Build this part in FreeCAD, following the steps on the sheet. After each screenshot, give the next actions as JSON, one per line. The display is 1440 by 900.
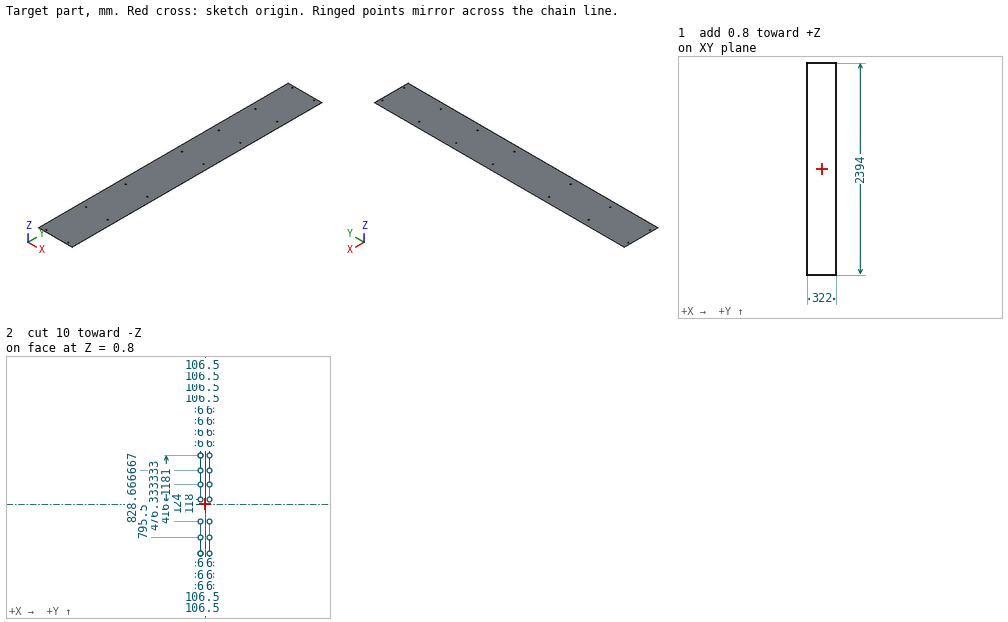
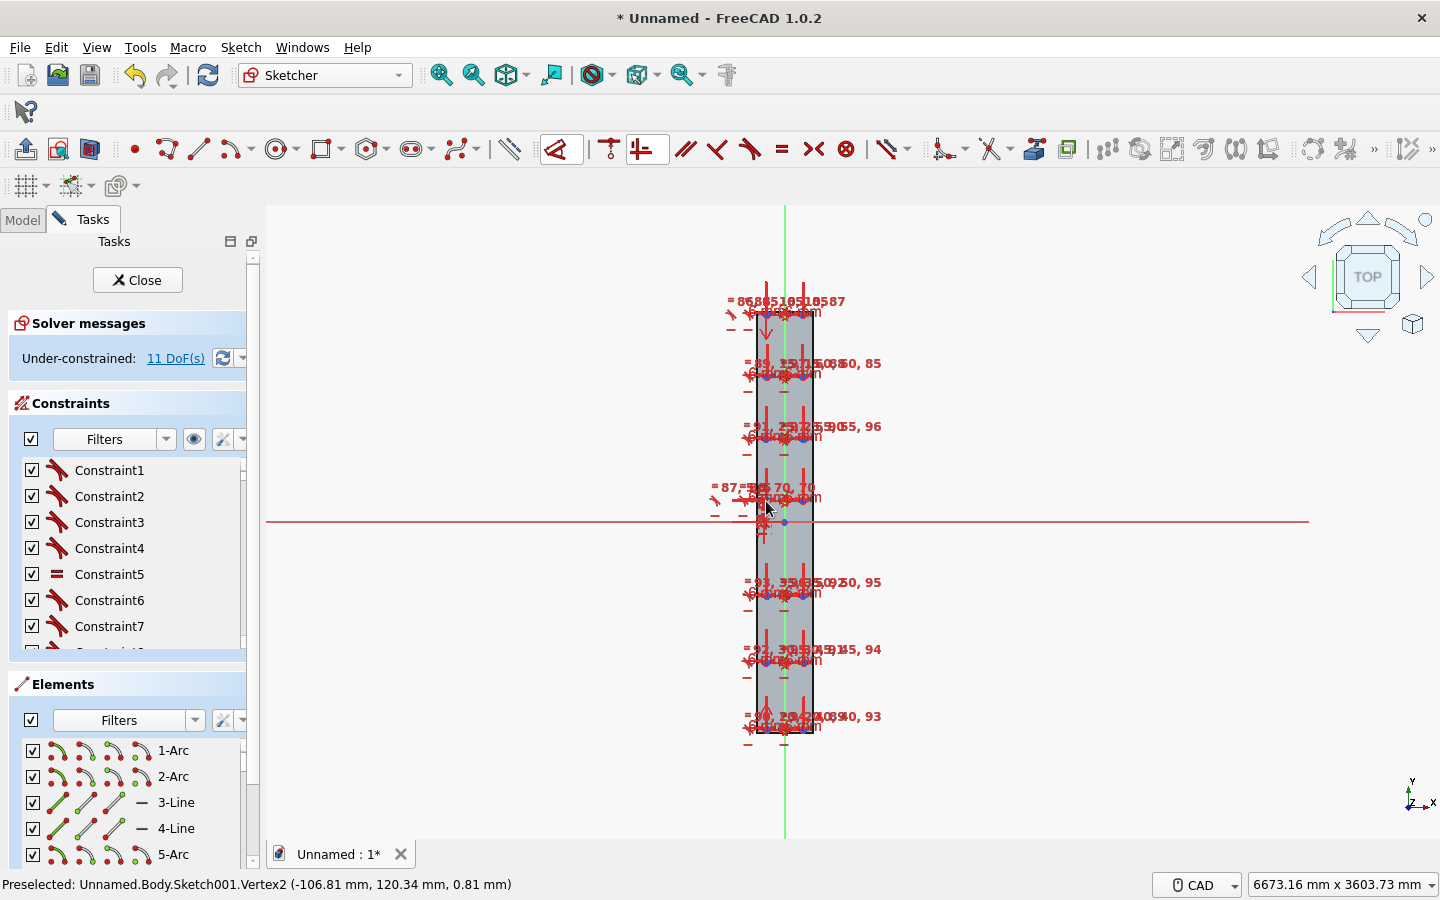
{"action": "scroll", "coordinate": [766, 595], "scroll_direction": "up", "scroll_amount": 14}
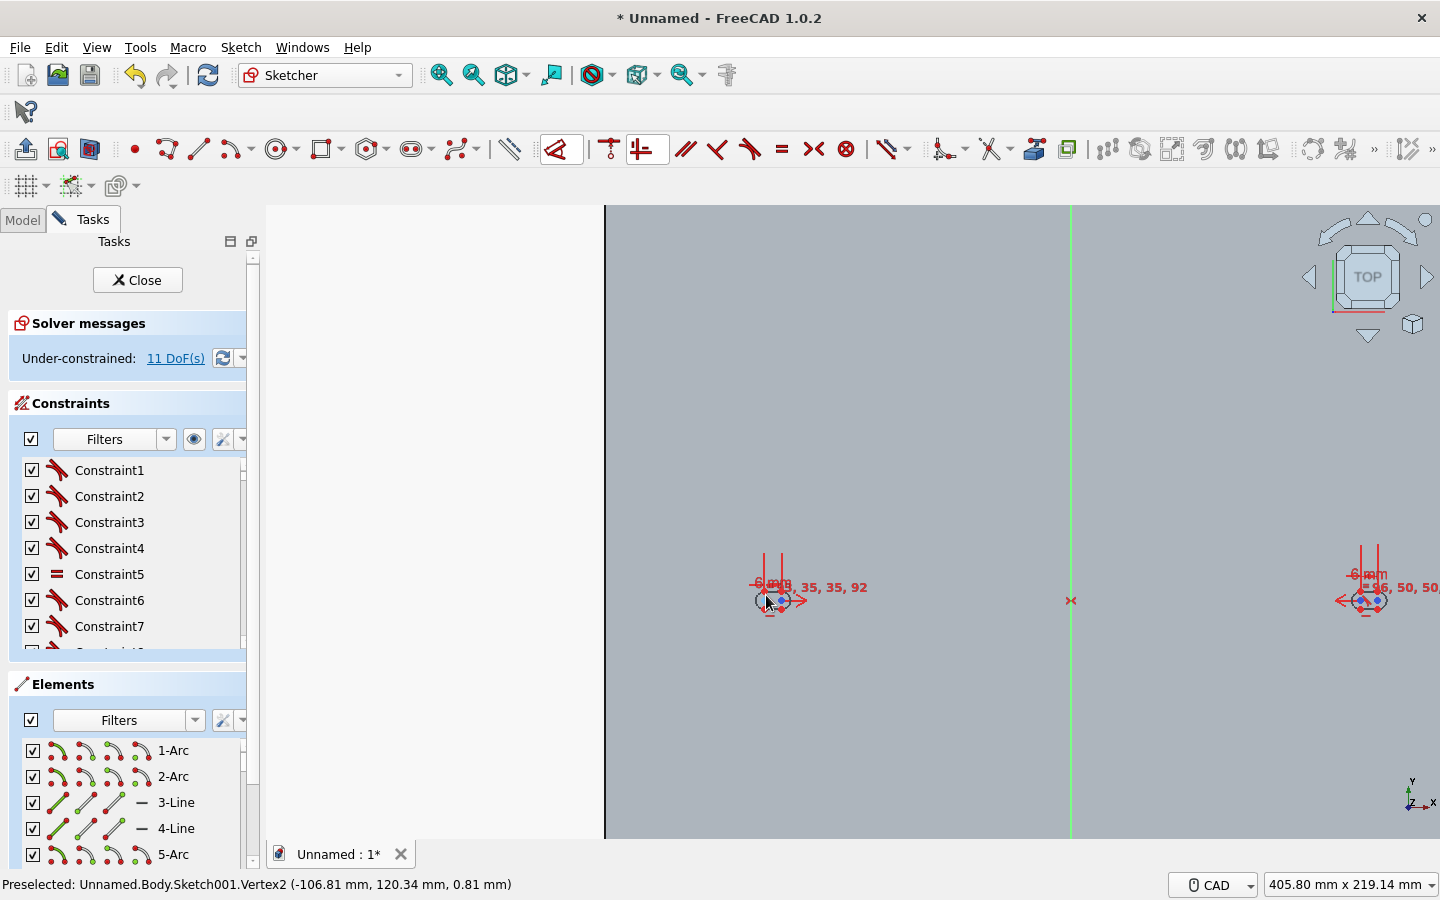
{"action": "left_click", "coordinate": [764, 592]}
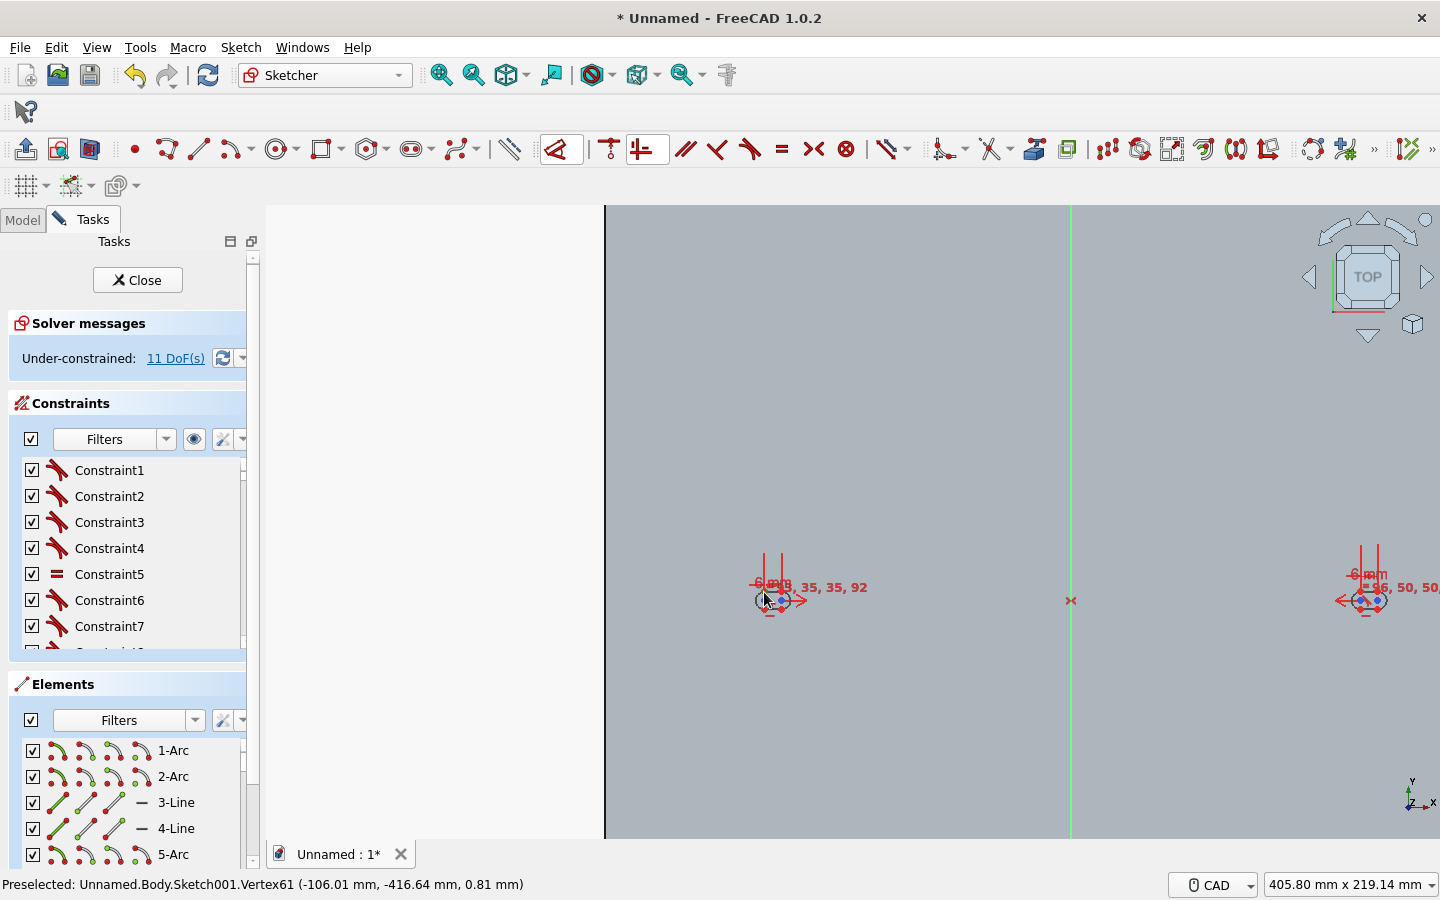
{"action": "left_click", "coordinate": [578, 150]}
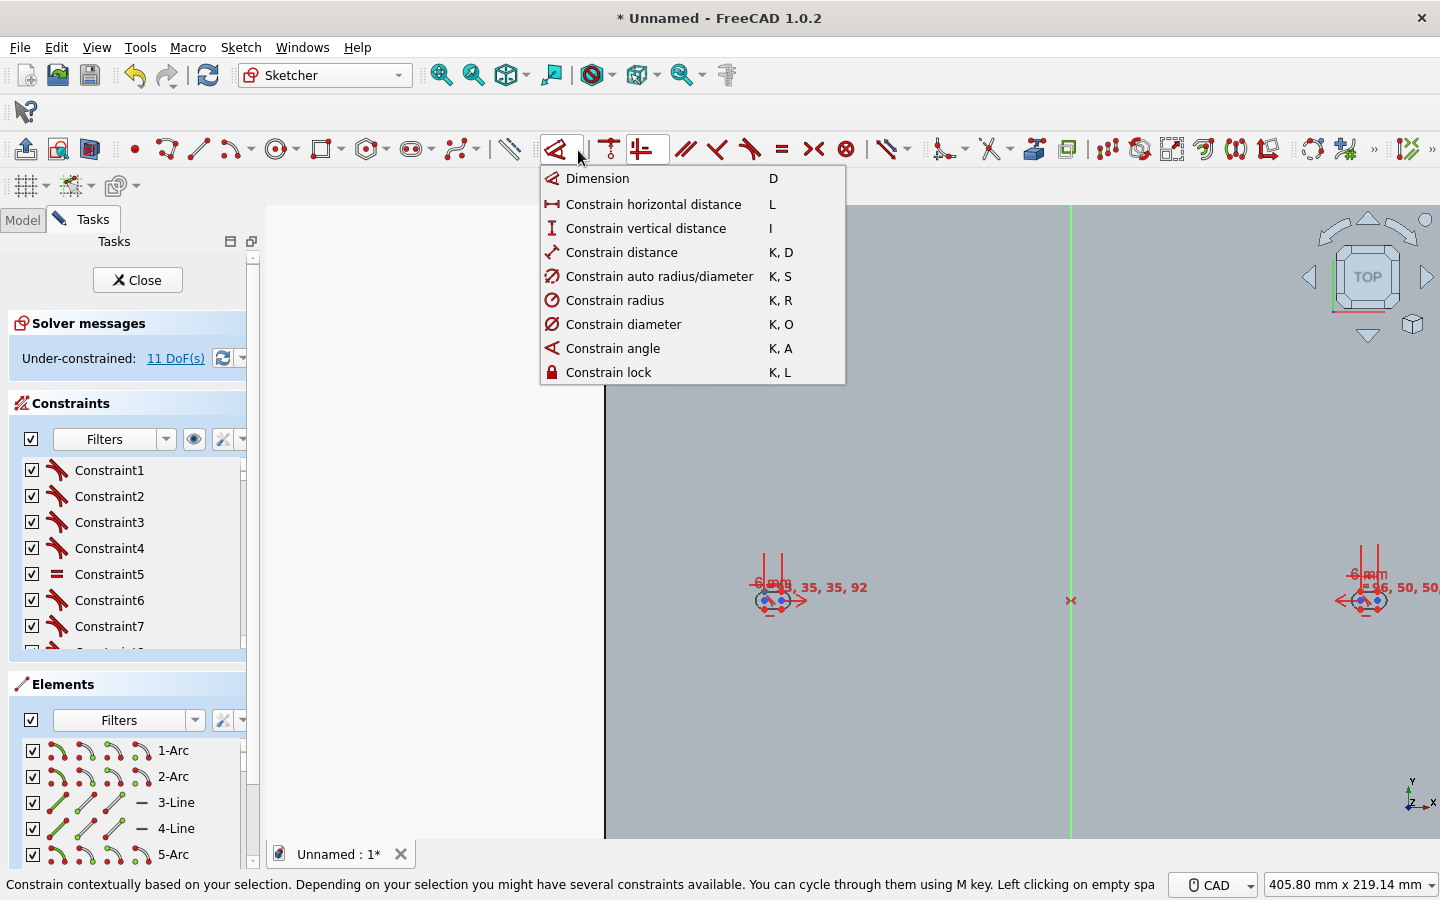
{"action": "left_click", "coordinate": [693, 228]}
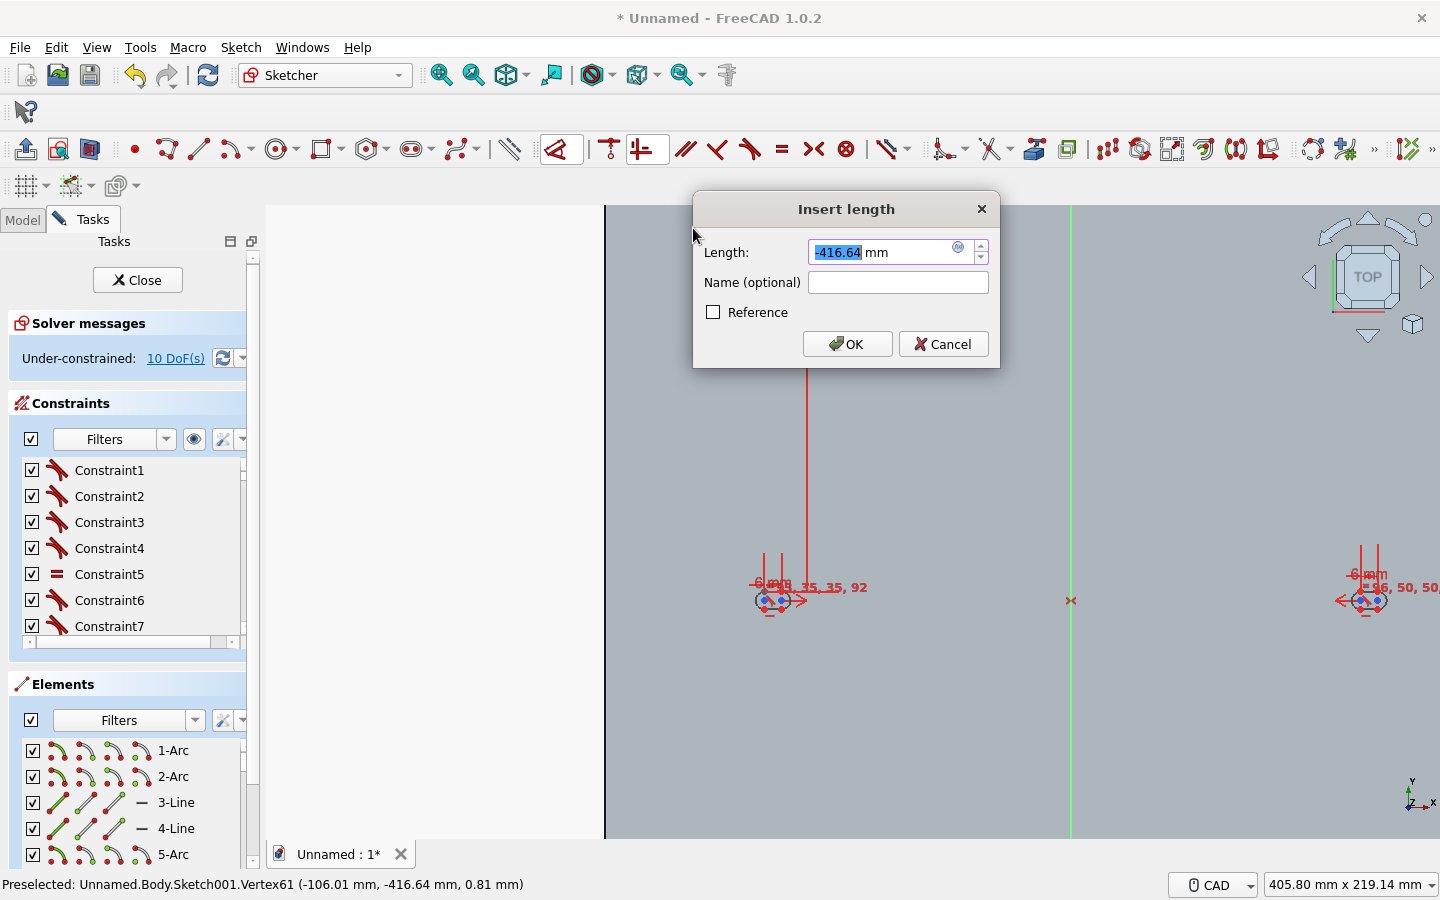
{"action": "type", "text": "-416"}
{"action": "key", "text": "Return"}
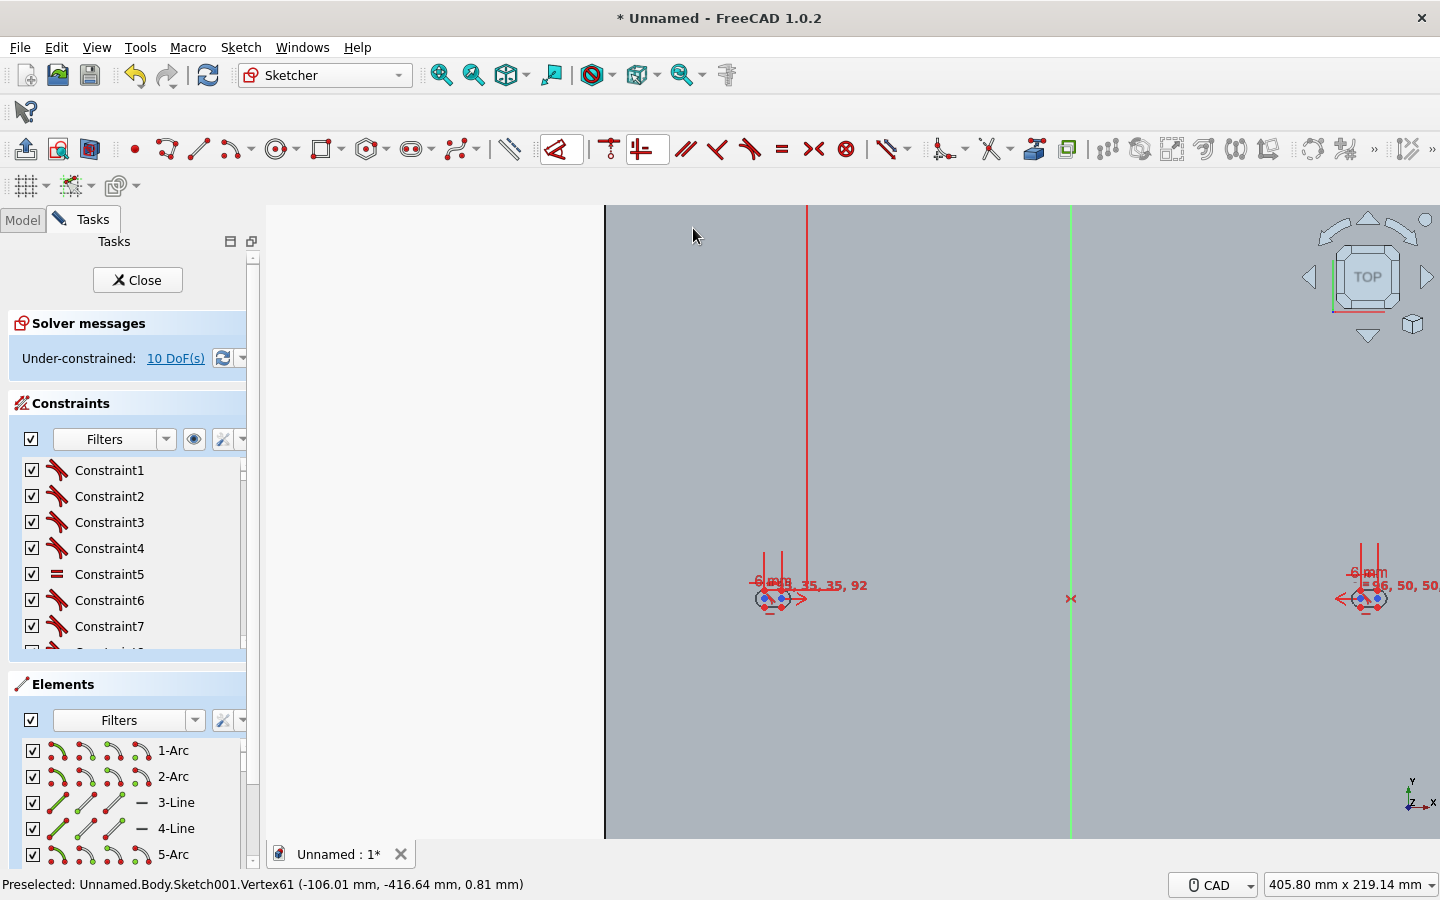
{"action": "scroll", "coordinate": [766, 596], "scroll_direction": "down", "scroll_amount": 14}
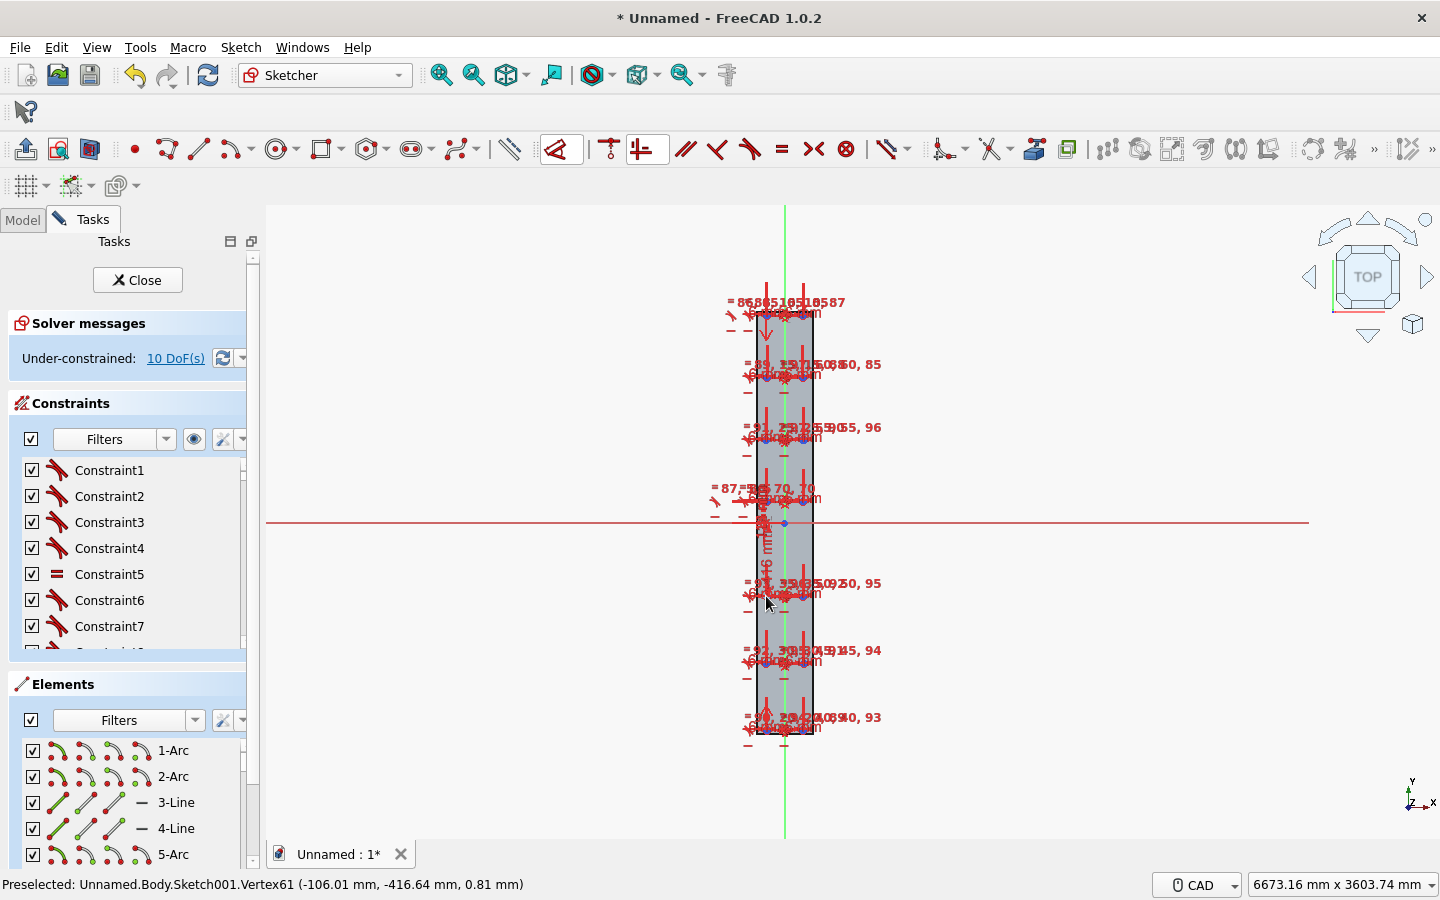
{"action": "scroll", "coordinate": [766, 315], "scroll_direction": "up", "scroll_amount": 14}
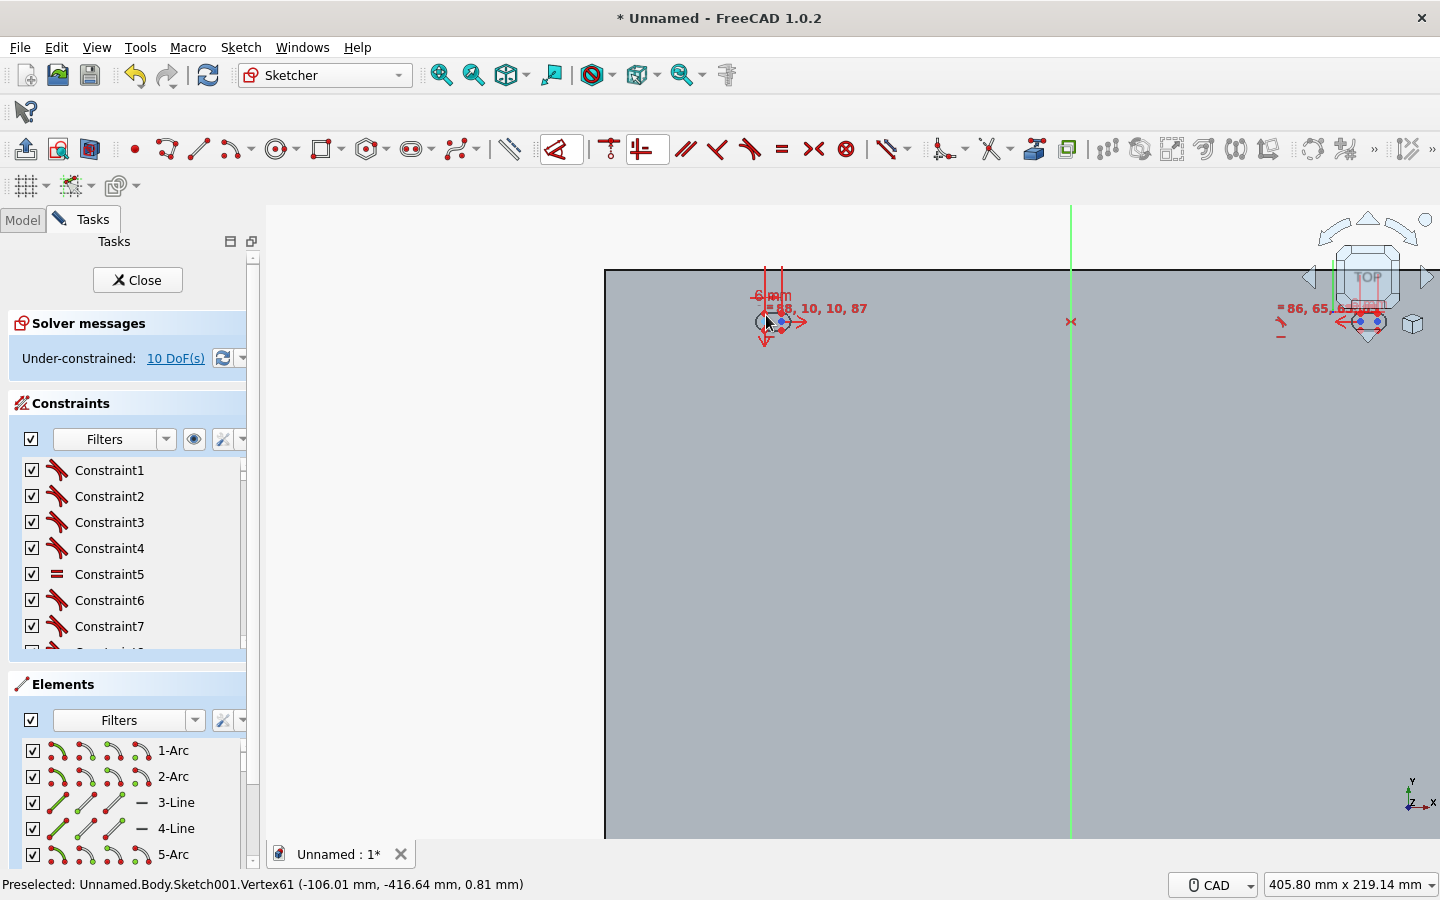
{"action": "left_click", "coordinate": [765, 313]}